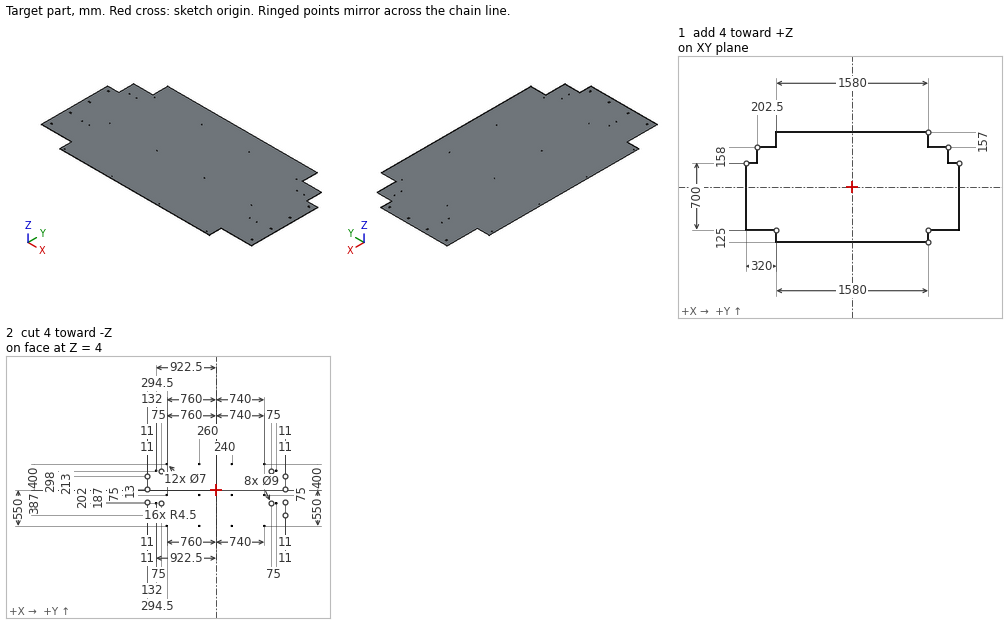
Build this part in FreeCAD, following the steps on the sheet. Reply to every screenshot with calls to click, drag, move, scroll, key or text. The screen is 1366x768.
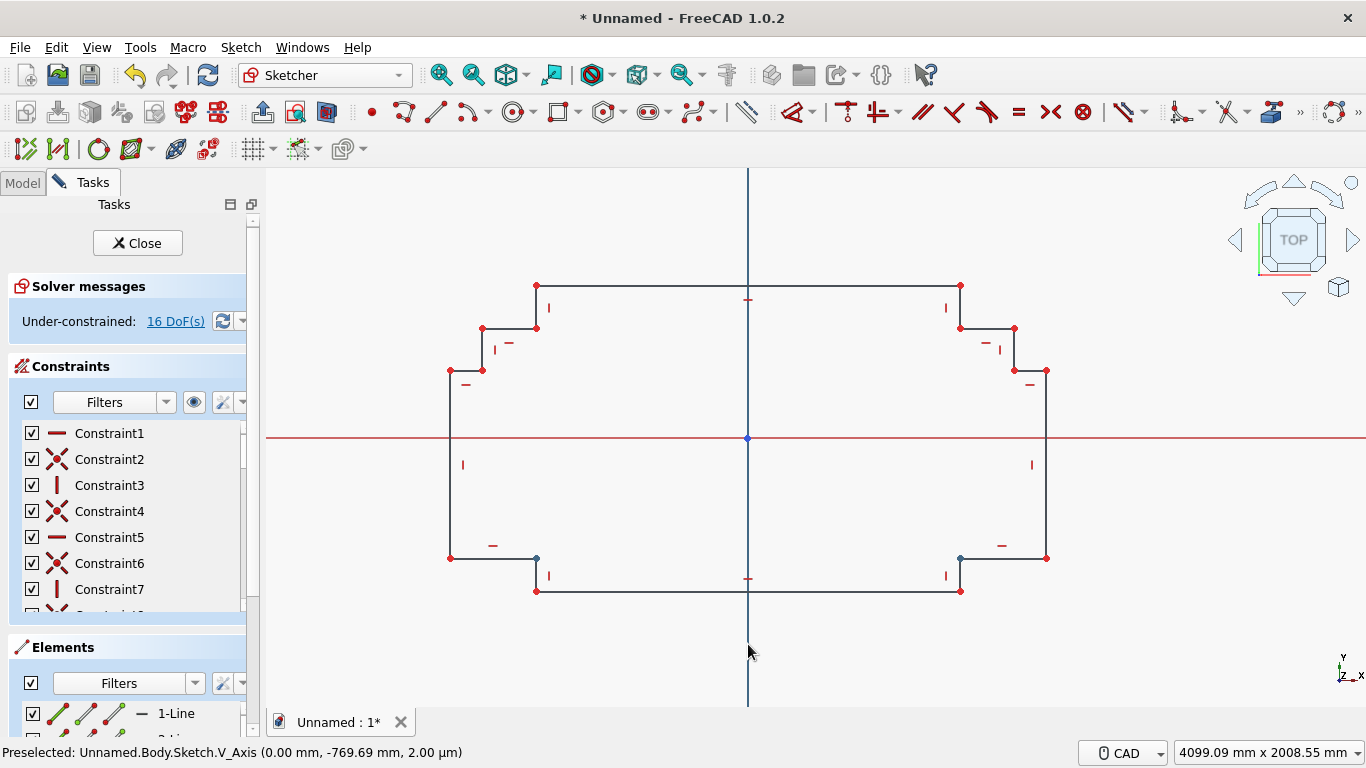
click(1052, 112)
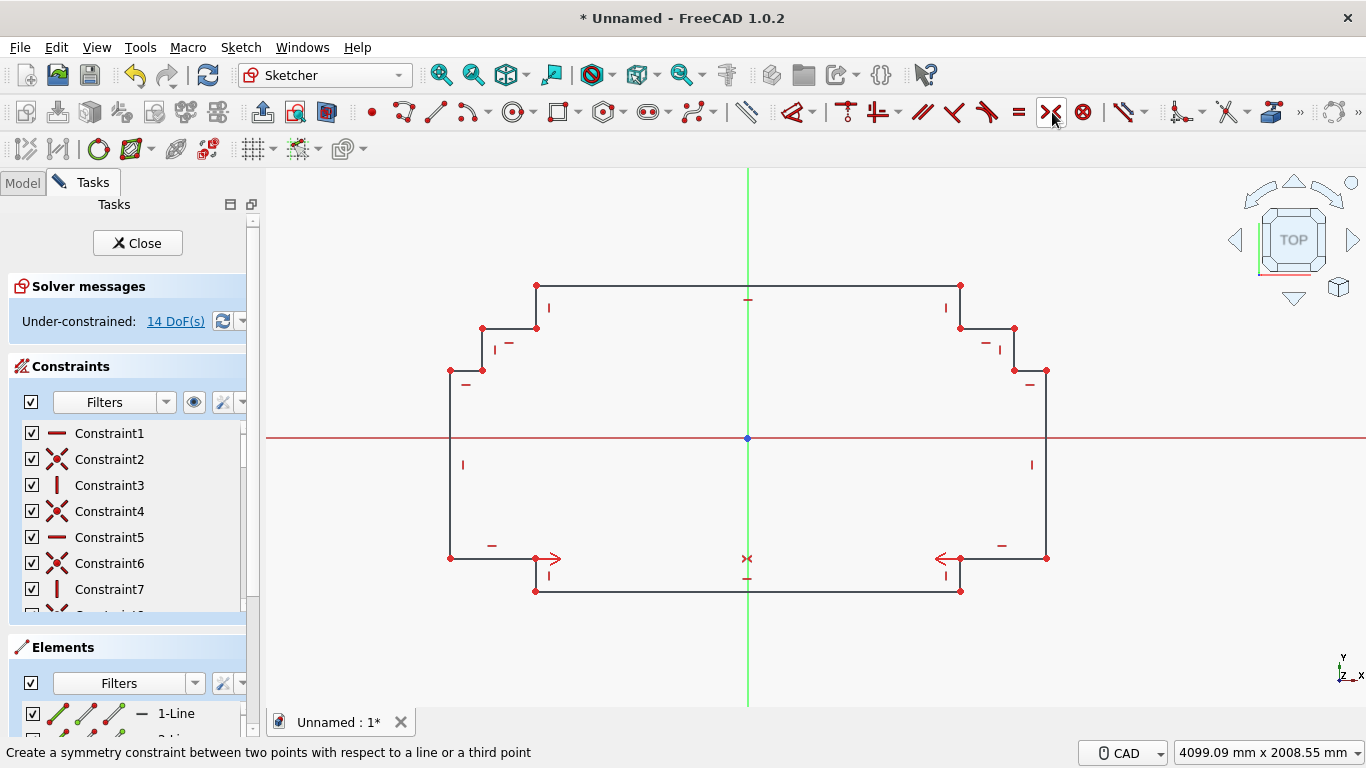
click(450, 371)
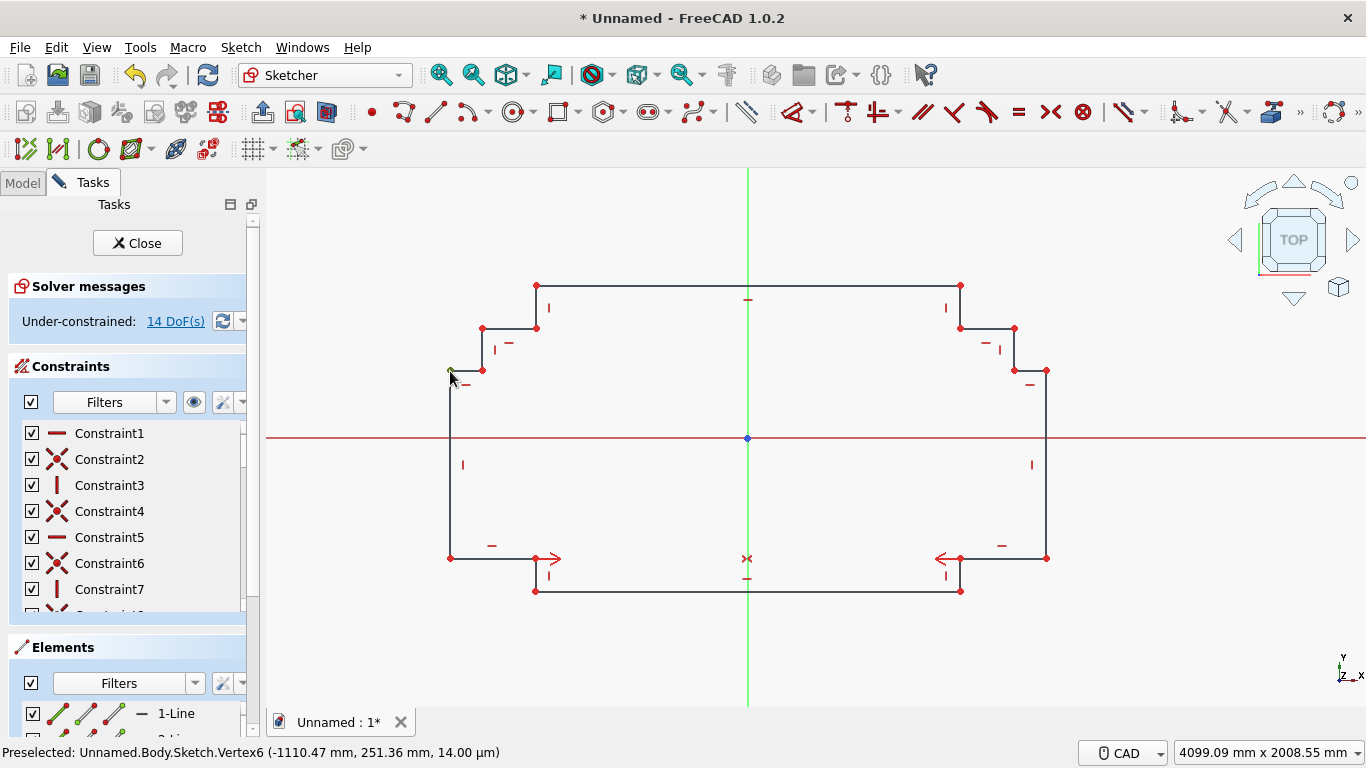
click(1046, 371)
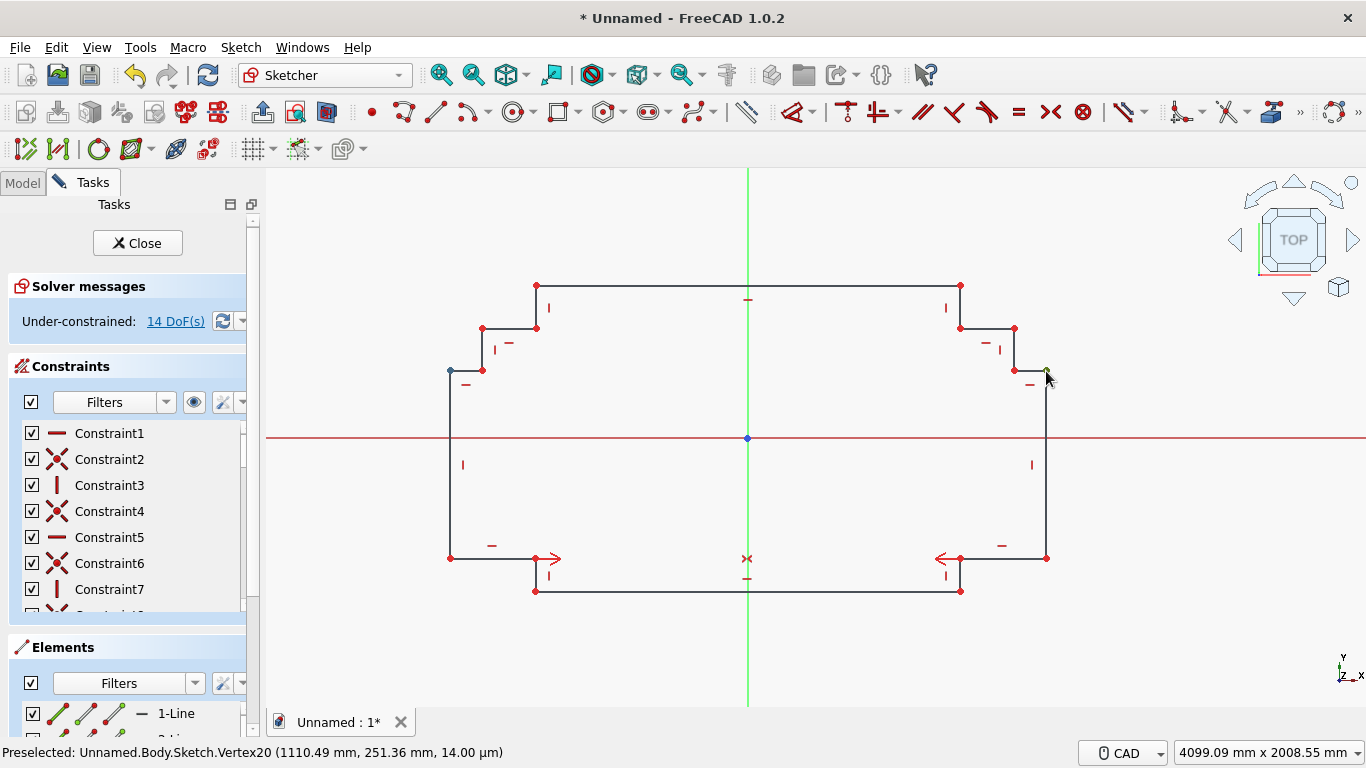
click(748, 644)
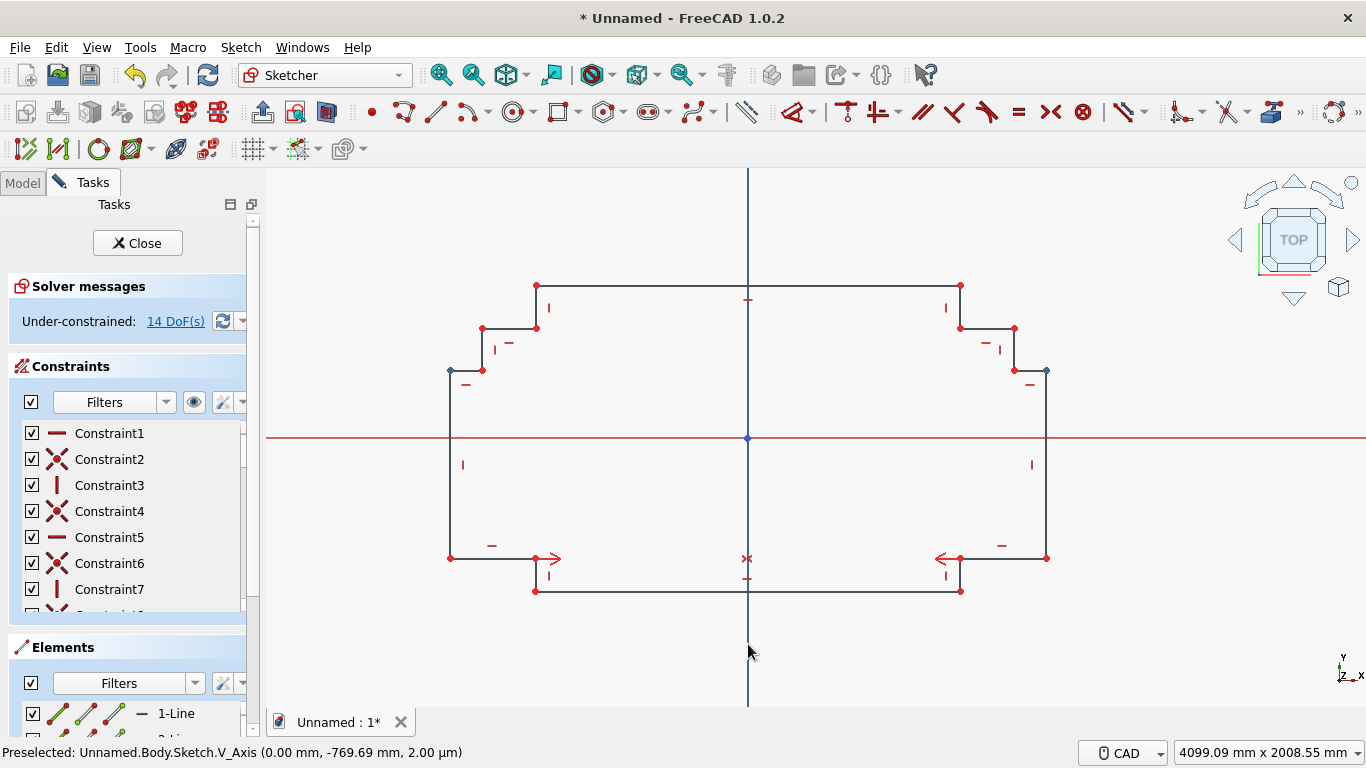
click(1052, 112)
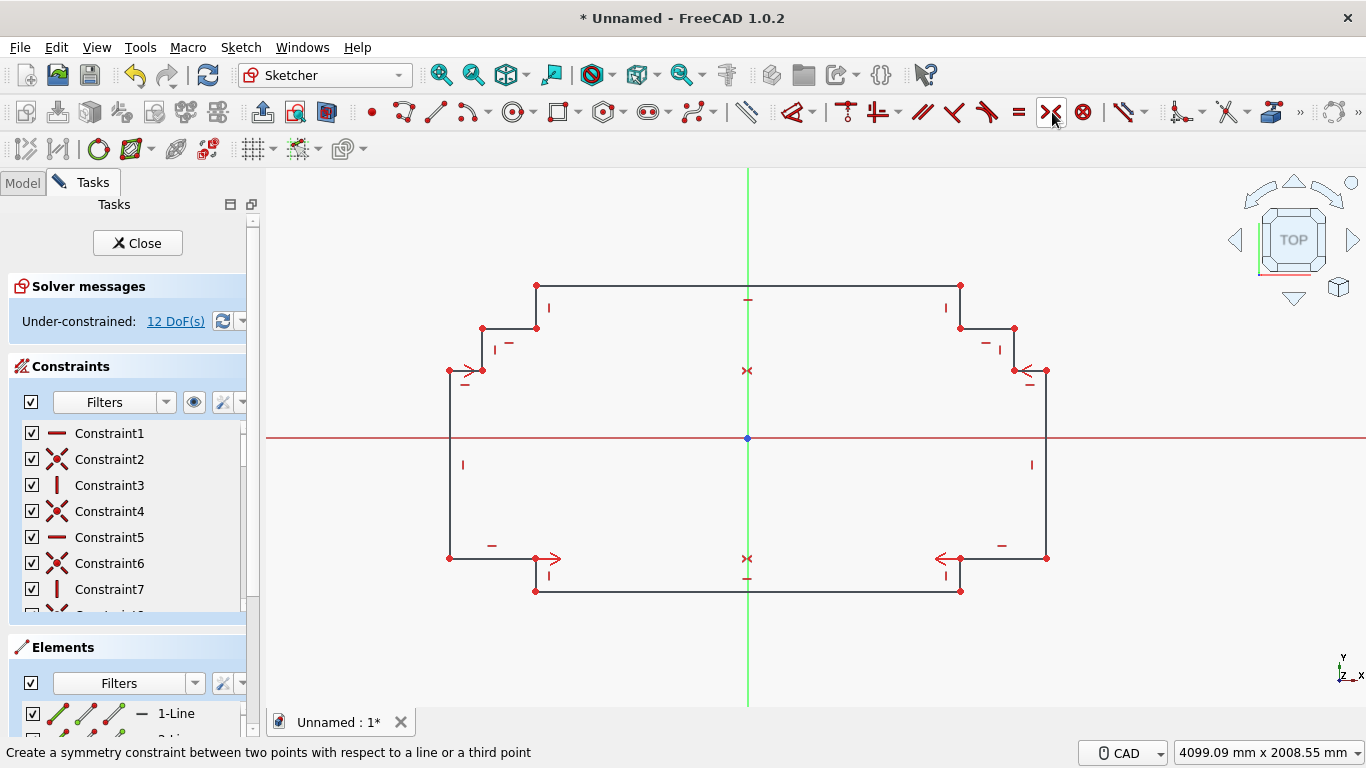
click(482, 329)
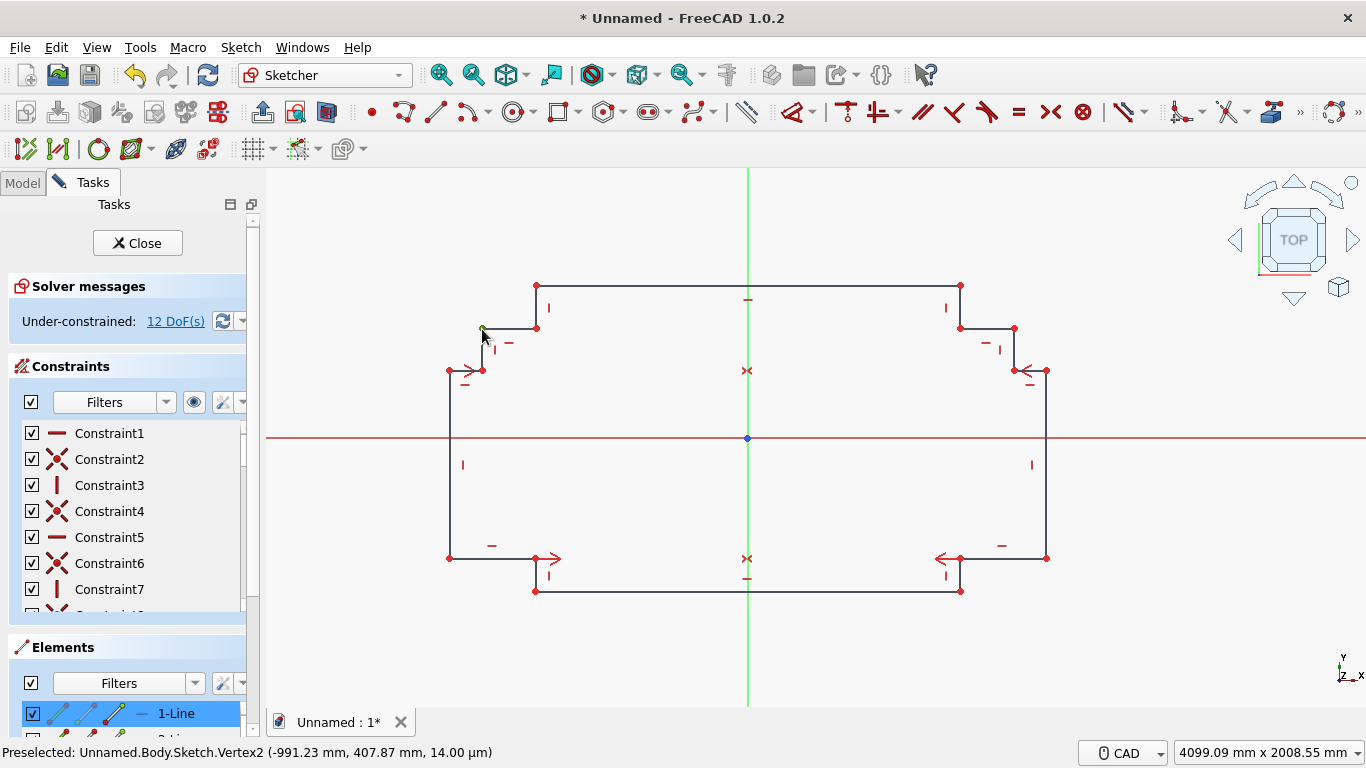
click(1014, 329)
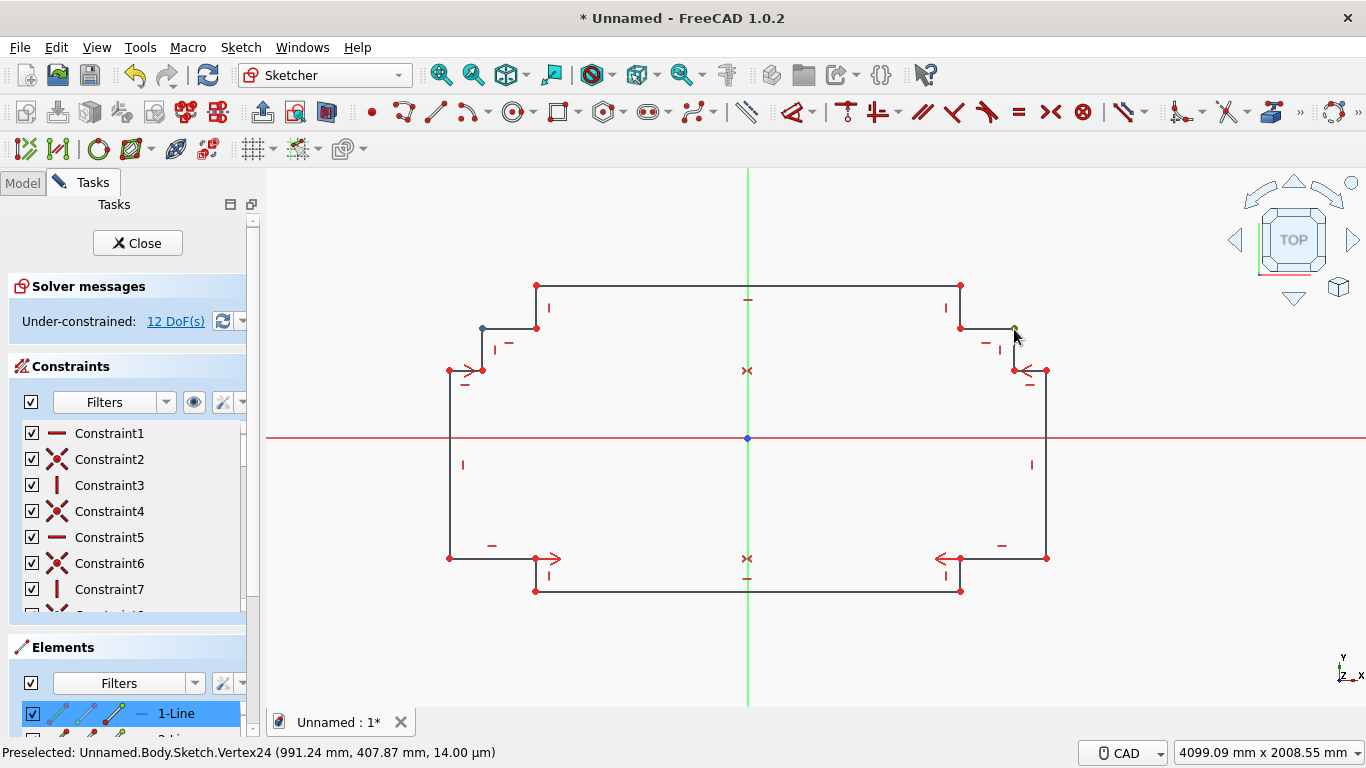
click(748, 644)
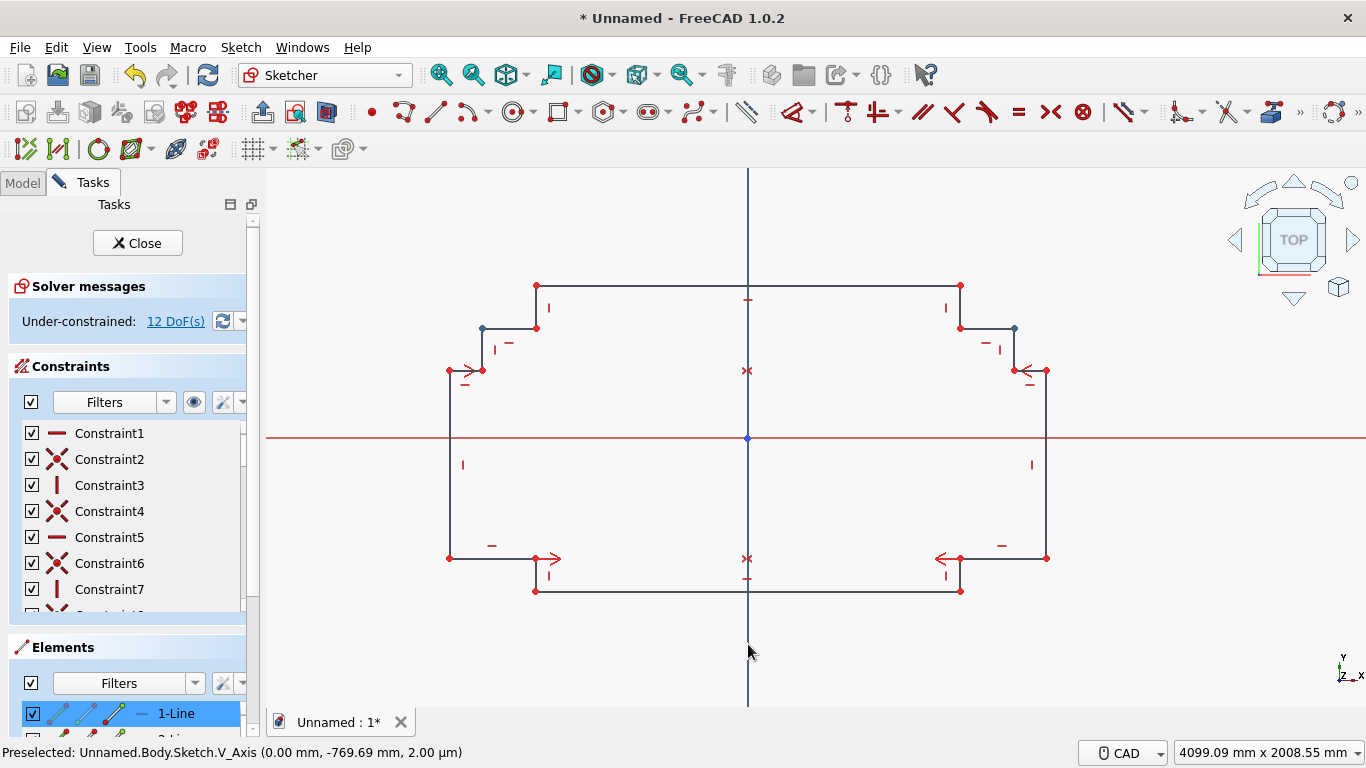
click(1052, 112)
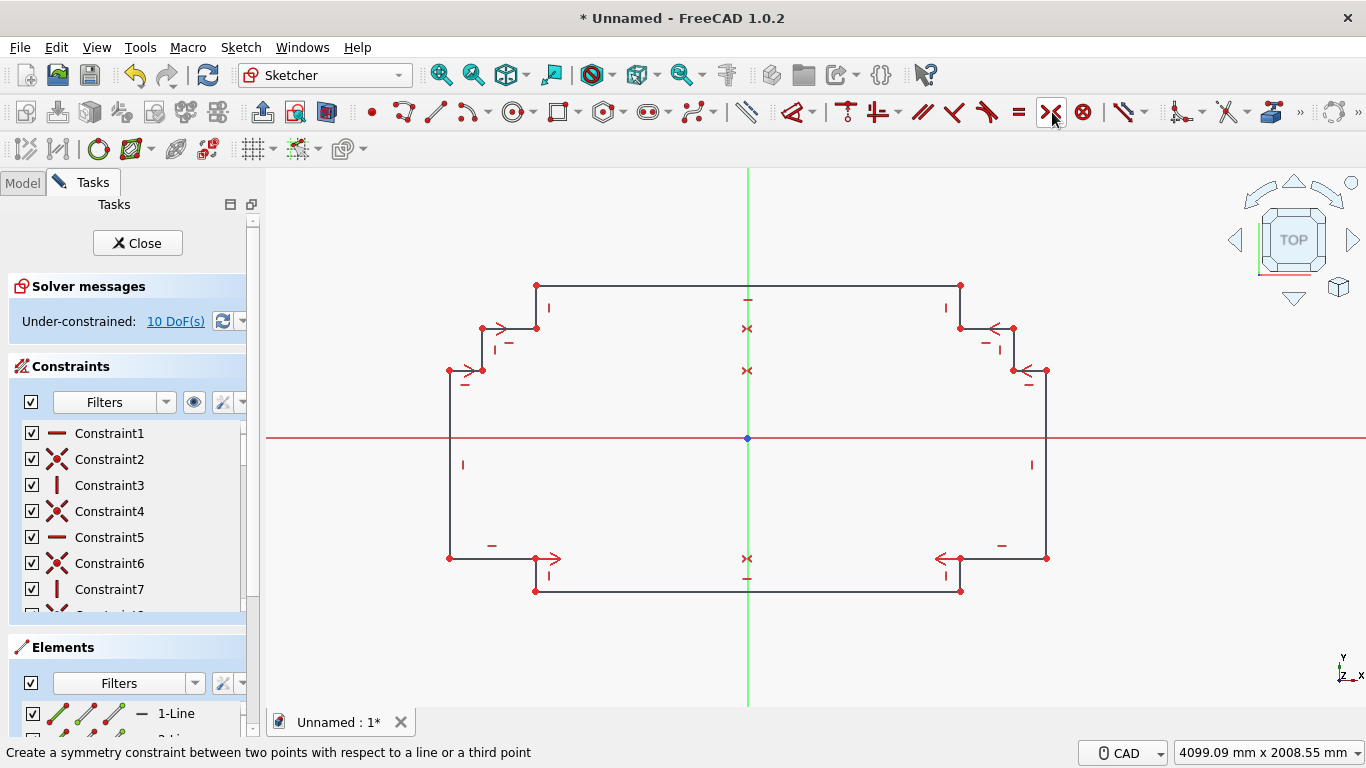
click(960, 592)